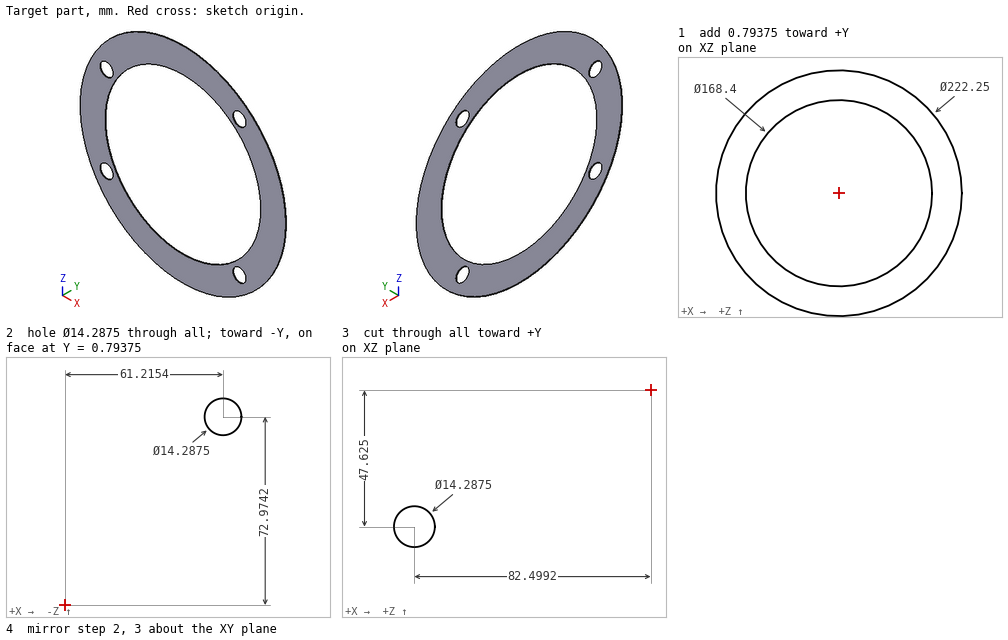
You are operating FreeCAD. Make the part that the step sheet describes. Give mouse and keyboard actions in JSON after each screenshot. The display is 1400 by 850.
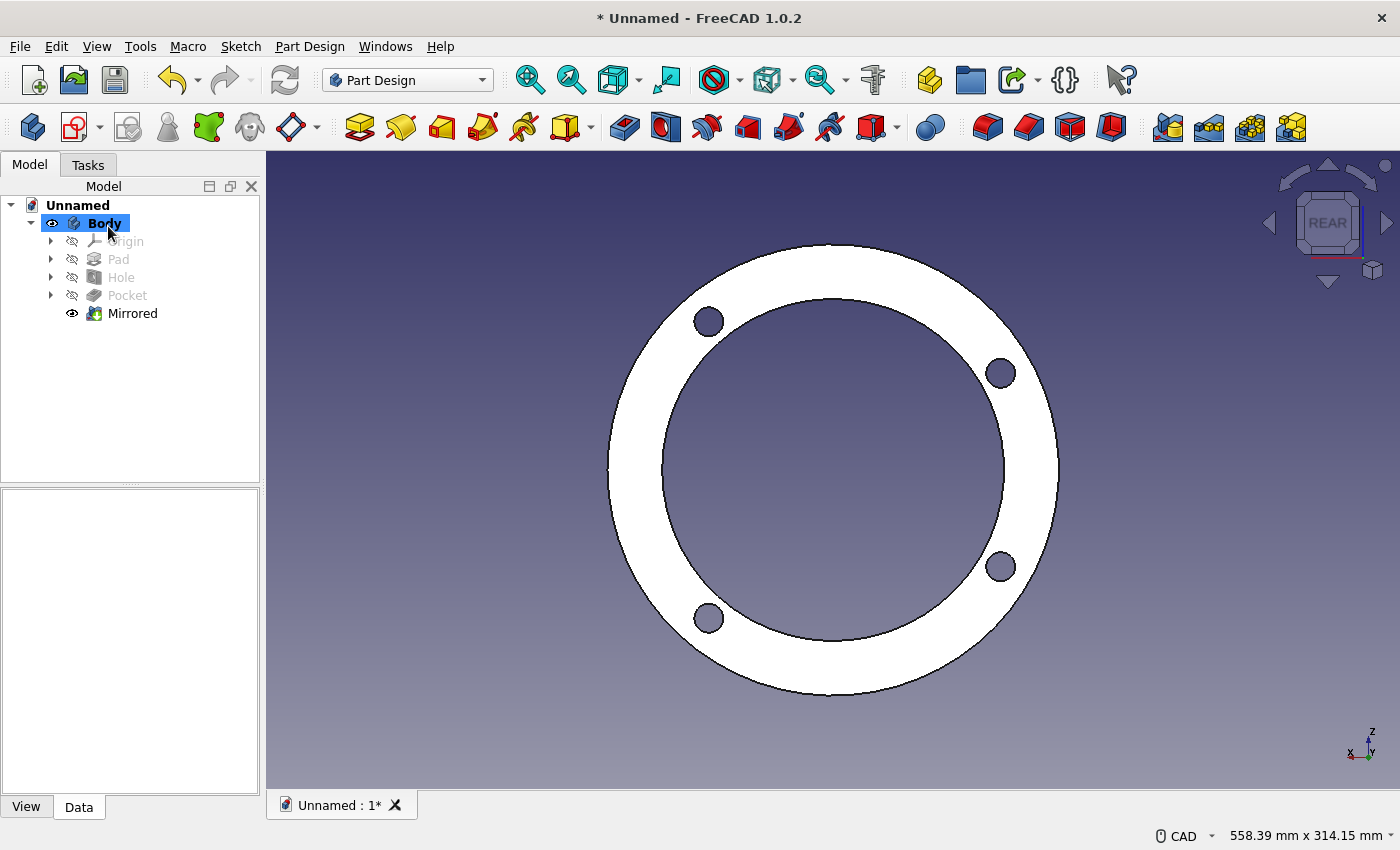
{"action": "key", "text": "0"}